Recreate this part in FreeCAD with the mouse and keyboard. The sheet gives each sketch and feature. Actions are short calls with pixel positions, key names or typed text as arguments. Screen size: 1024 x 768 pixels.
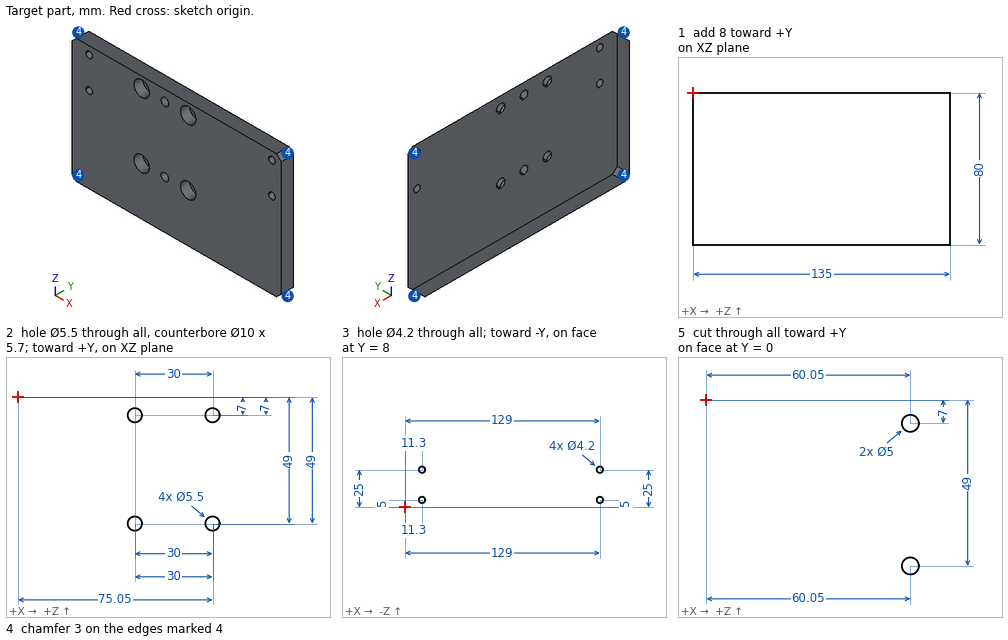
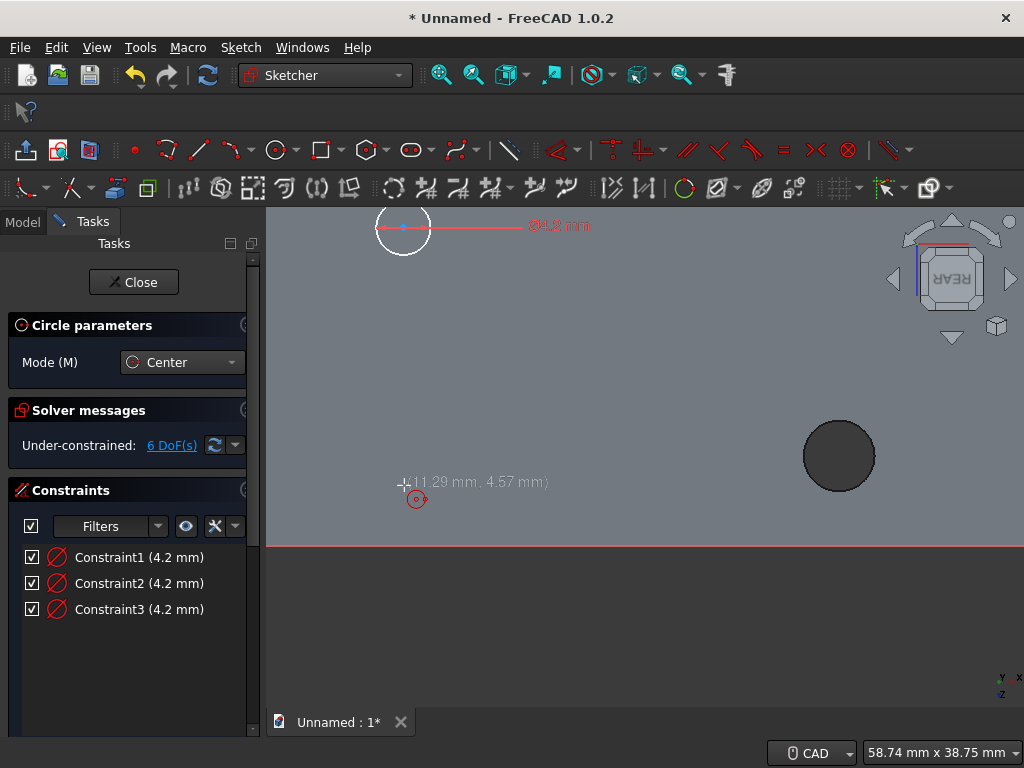
scroll(404, 485, down, 7)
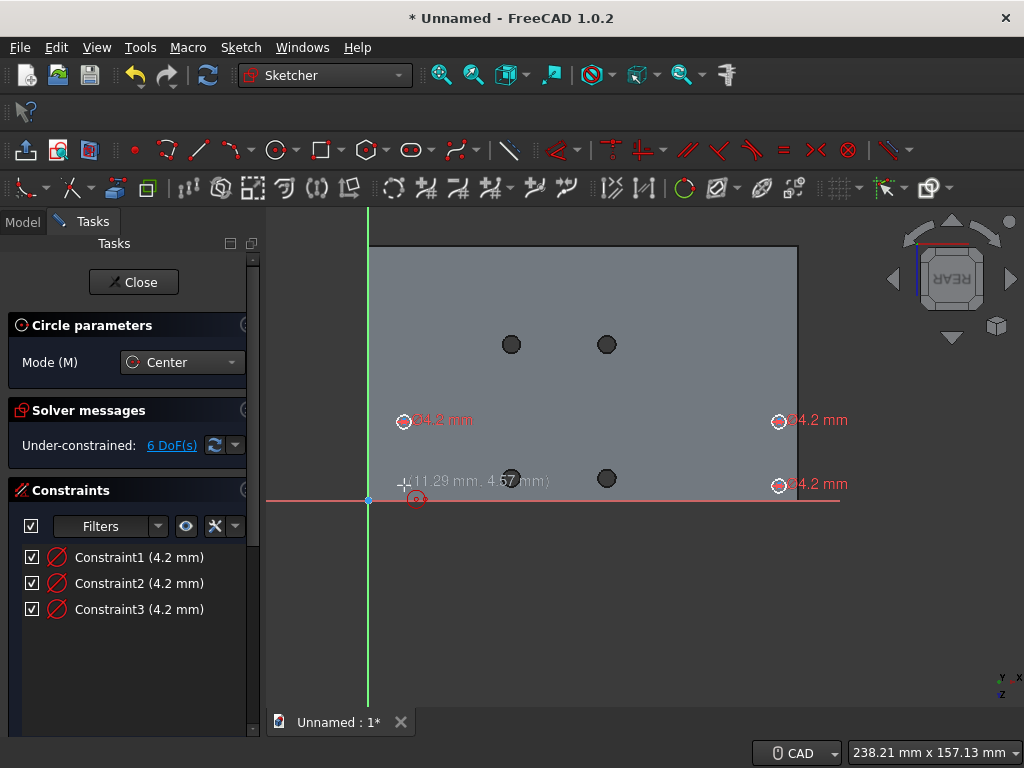
click(404, 485)
move(409, 480)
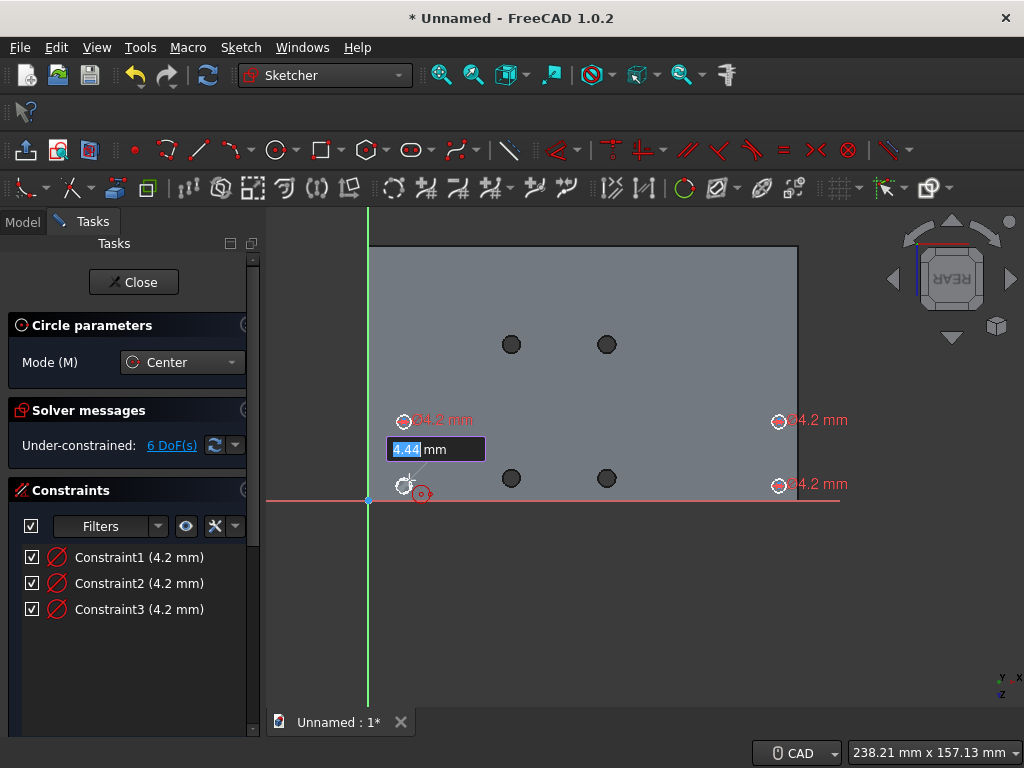
text(4.2)
key(Return)
key(Escape)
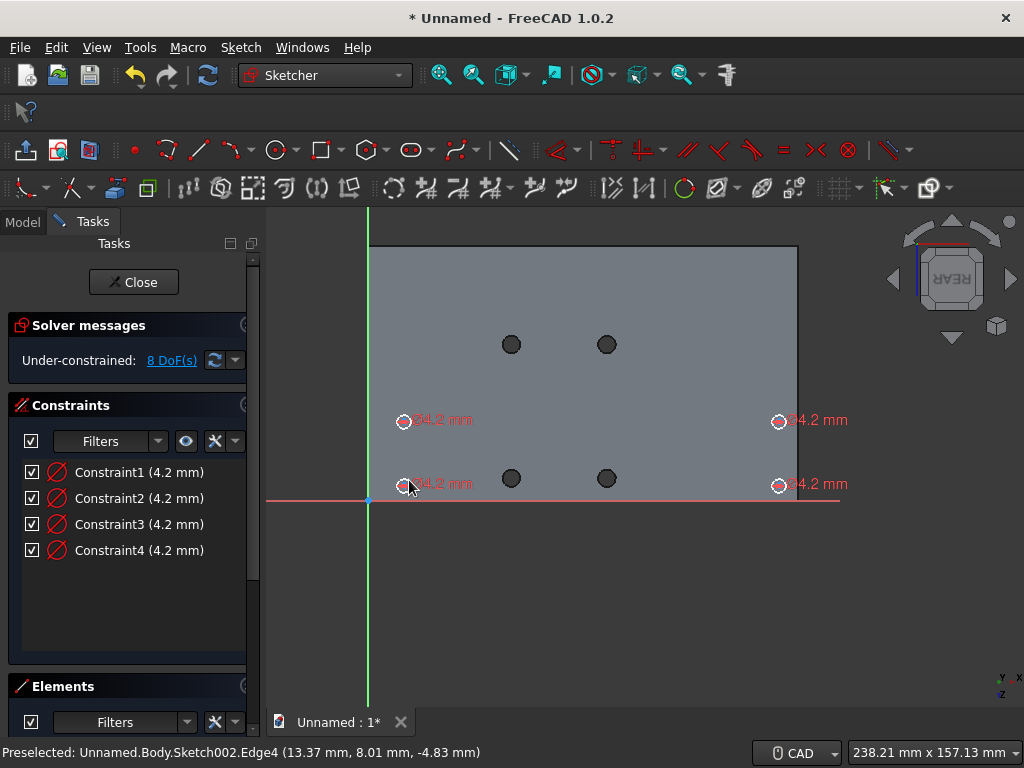
scroll(779, 486, up, 5)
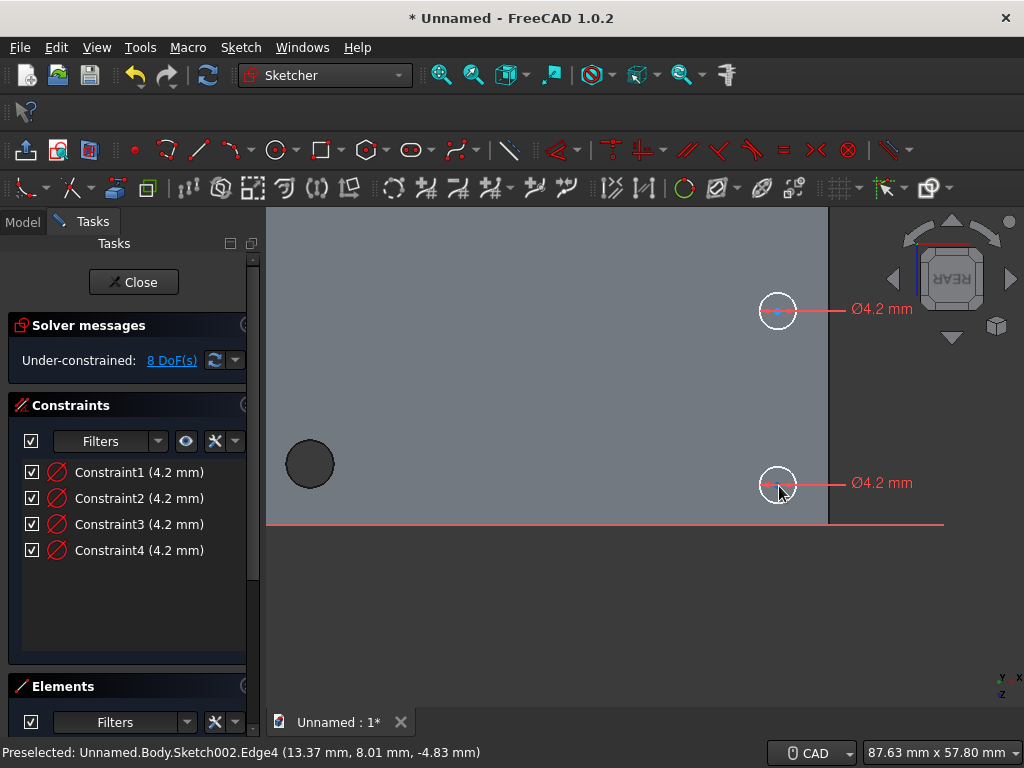
click(778, 485)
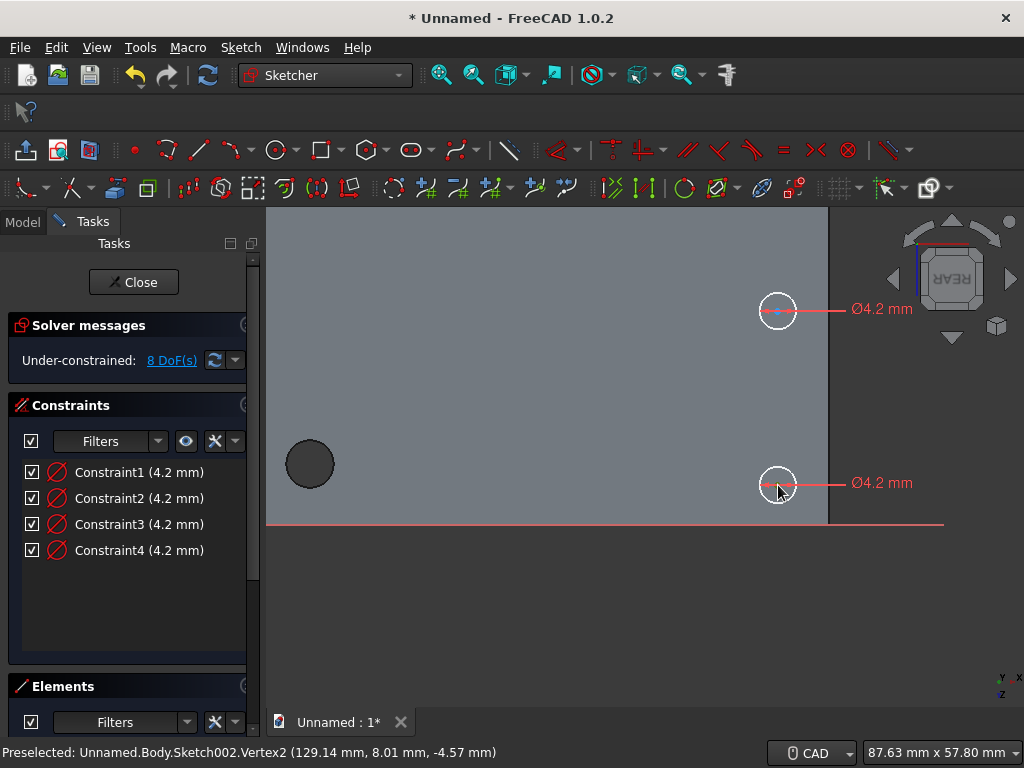
click(580, 150)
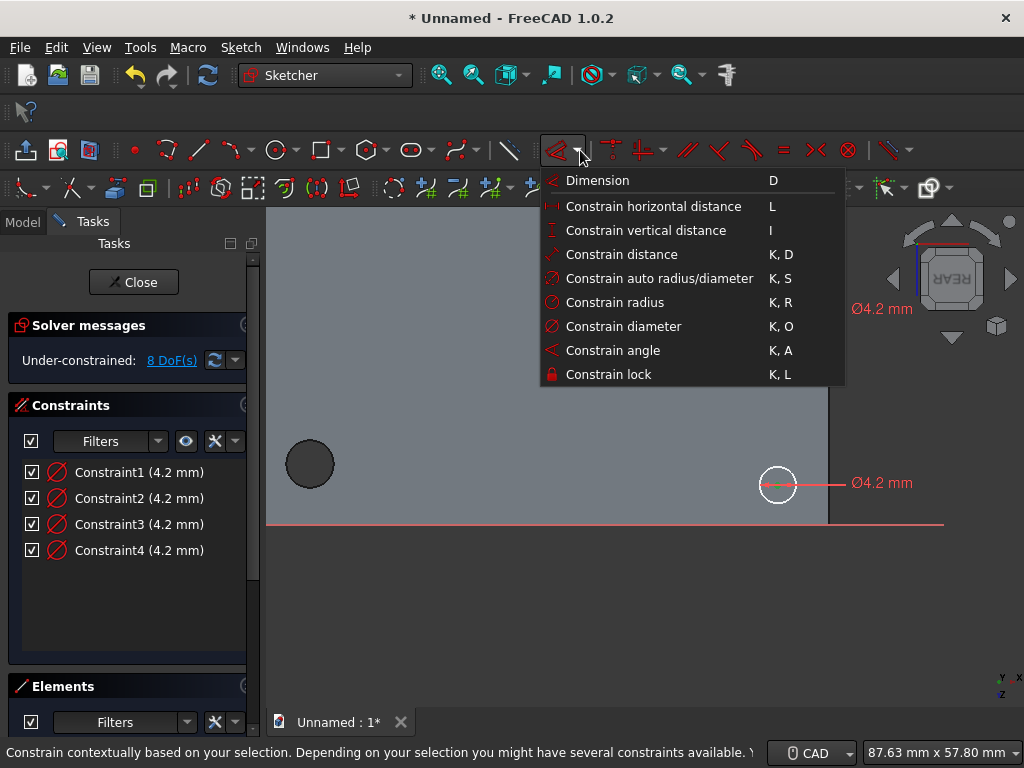
click(693, 230)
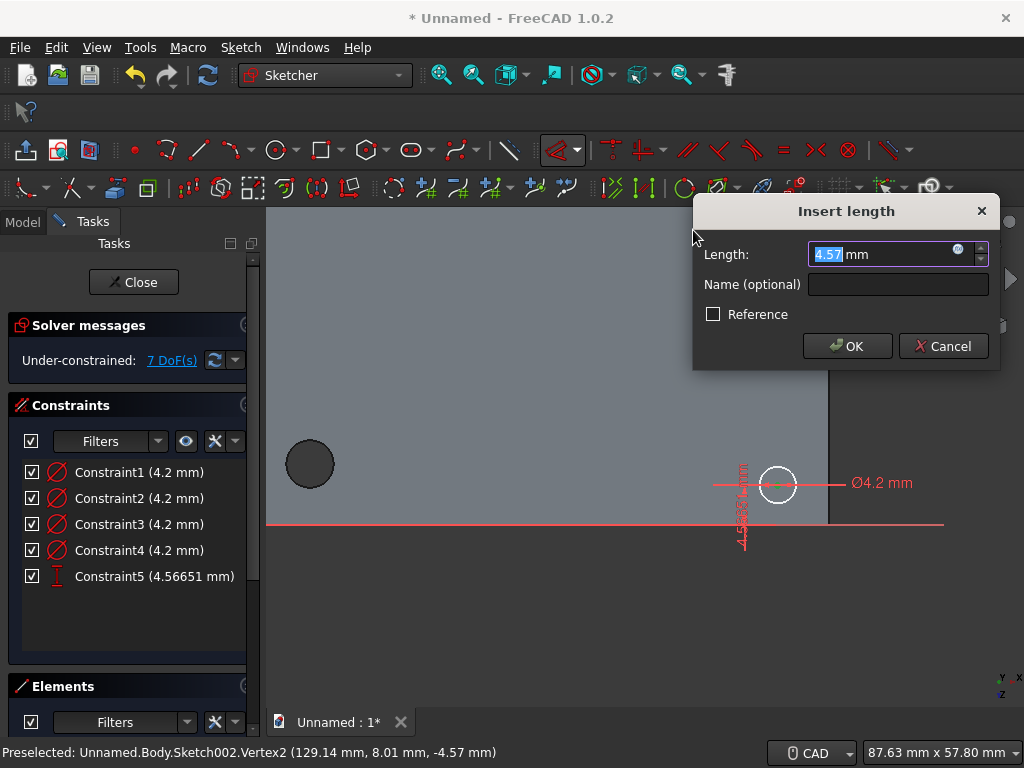
text(5)
key(Return)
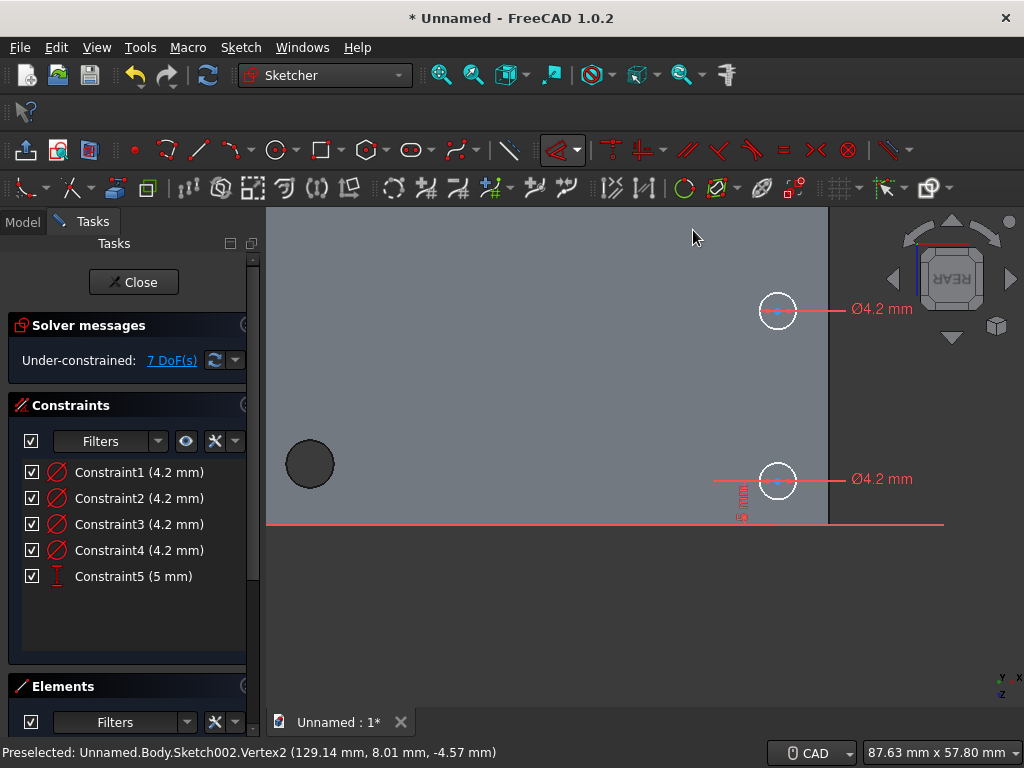
scroll(779, 486, down, 5)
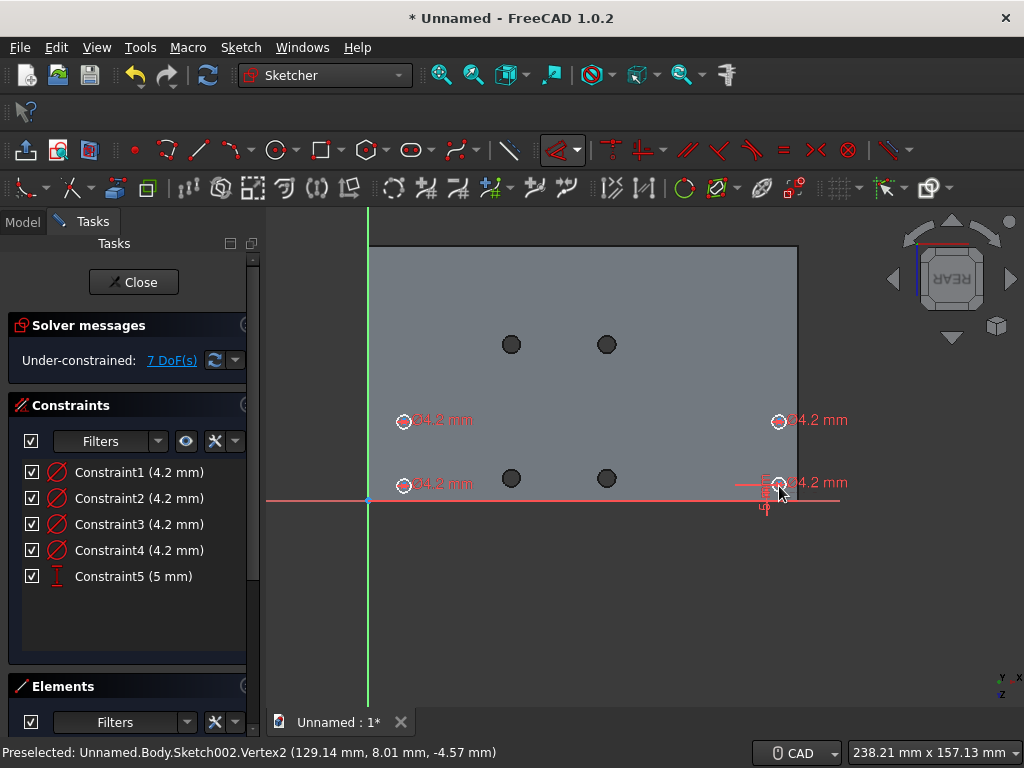
scroll(404, 486, up, 5)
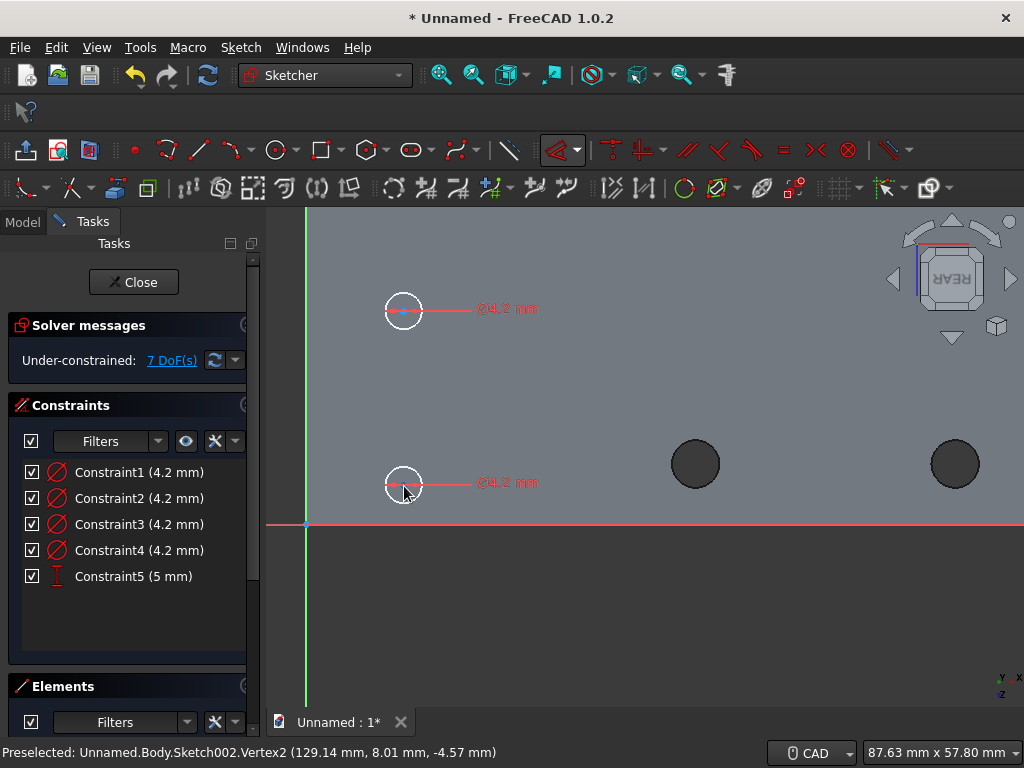
click(404, 485)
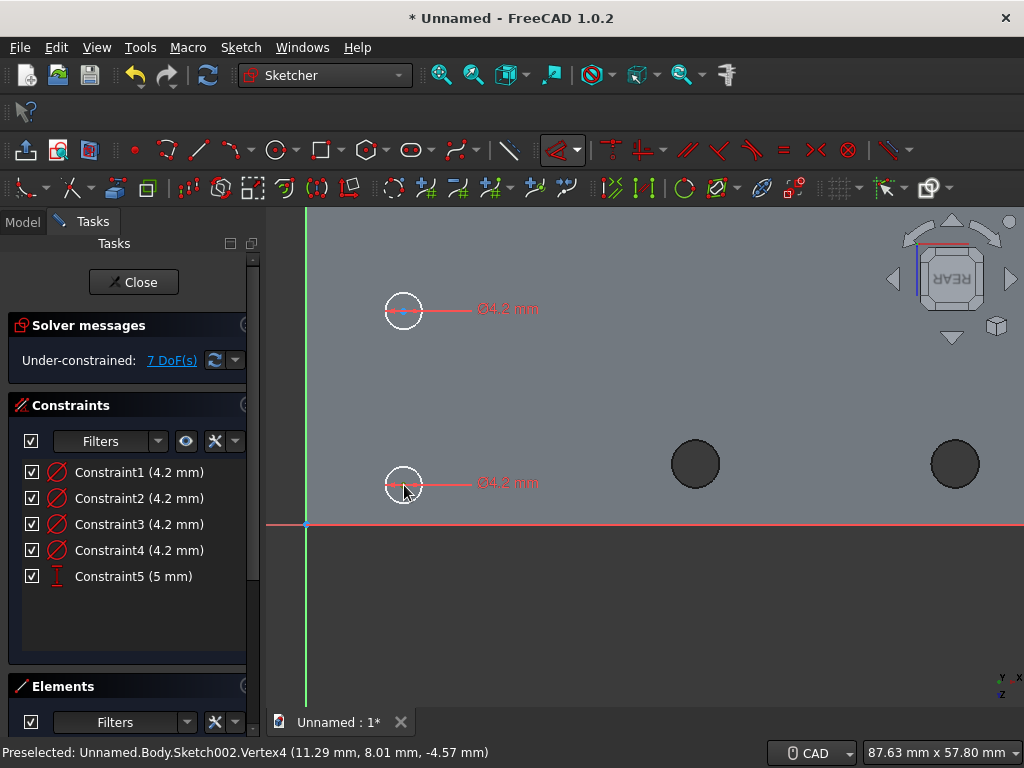
key(i)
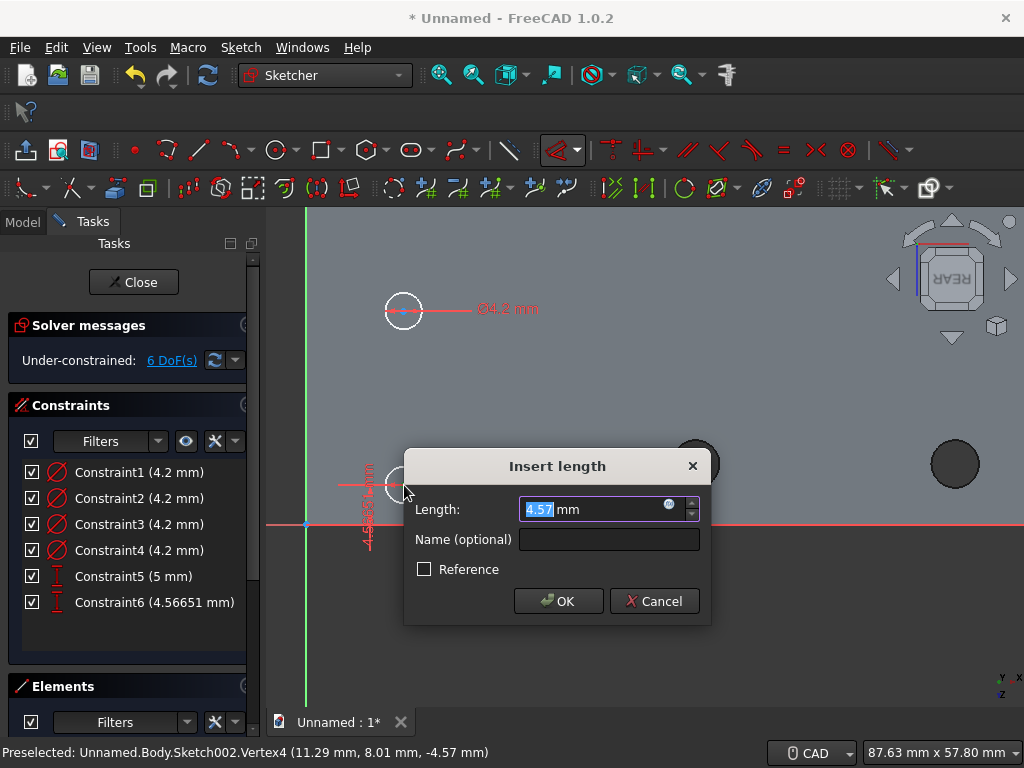
text(5)
key(Return)